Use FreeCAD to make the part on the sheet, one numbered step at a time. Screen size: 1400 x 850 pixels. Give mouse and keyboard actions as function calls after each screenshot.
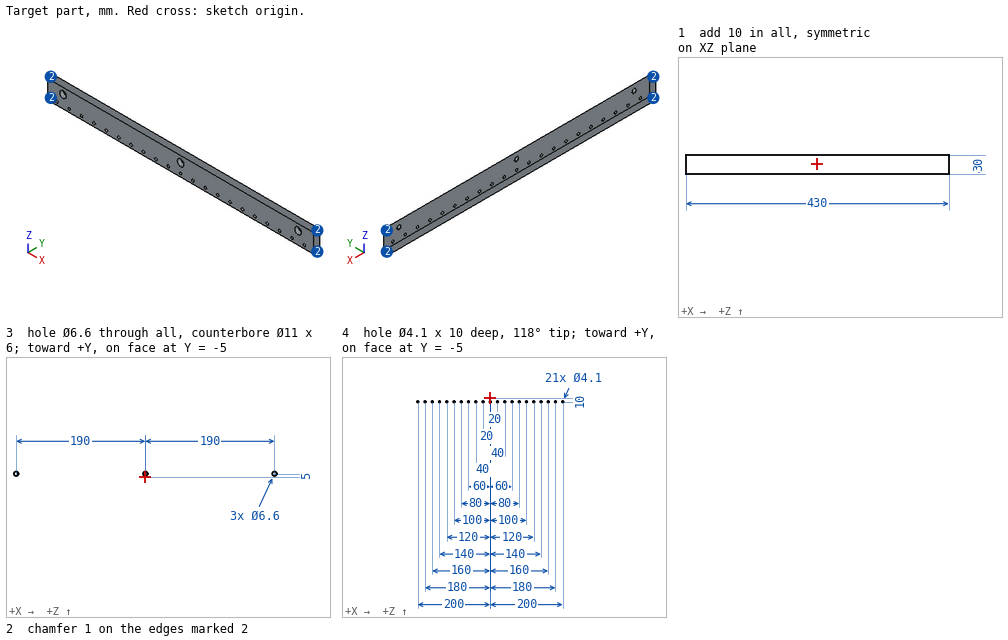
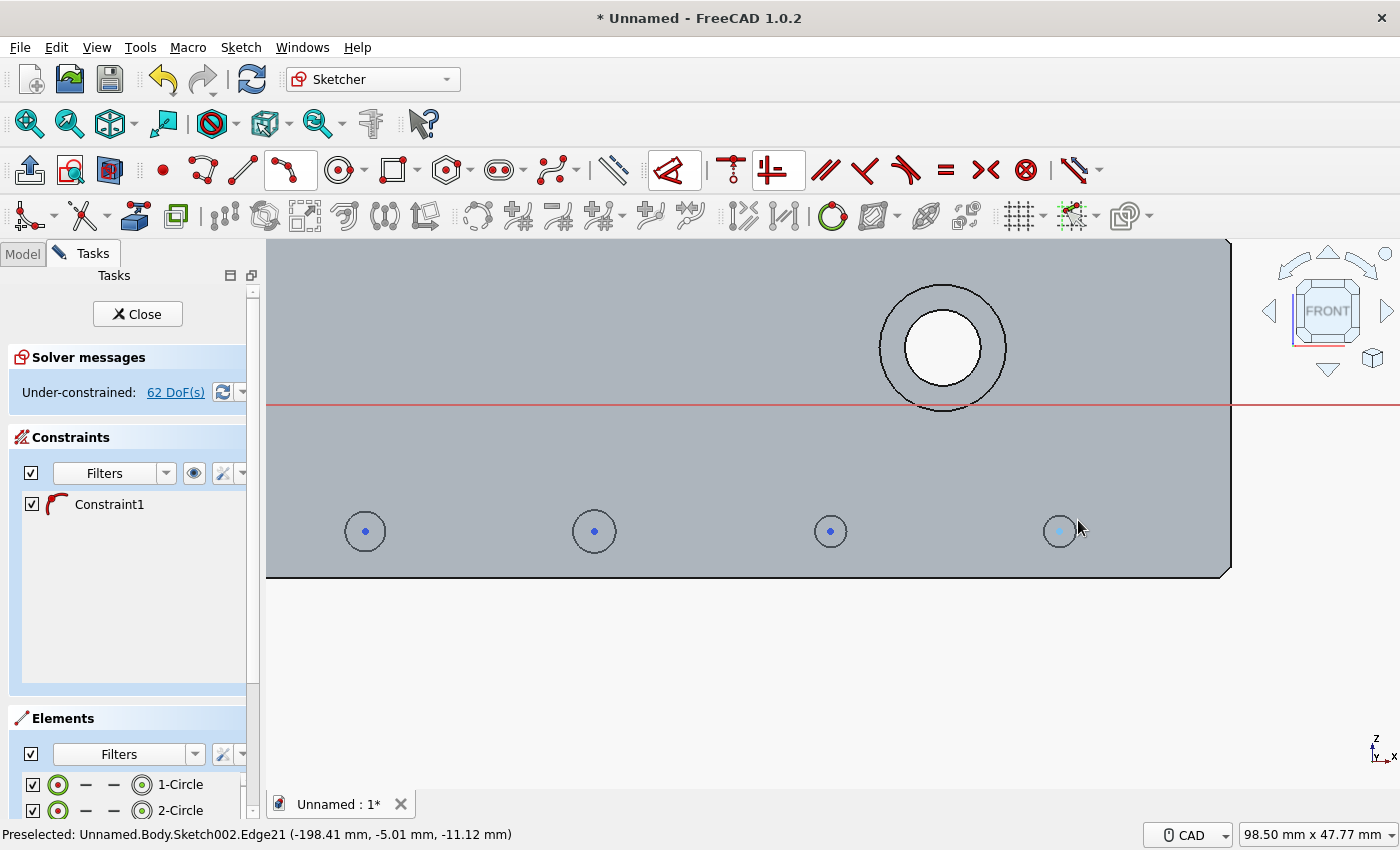
click(1071, 520)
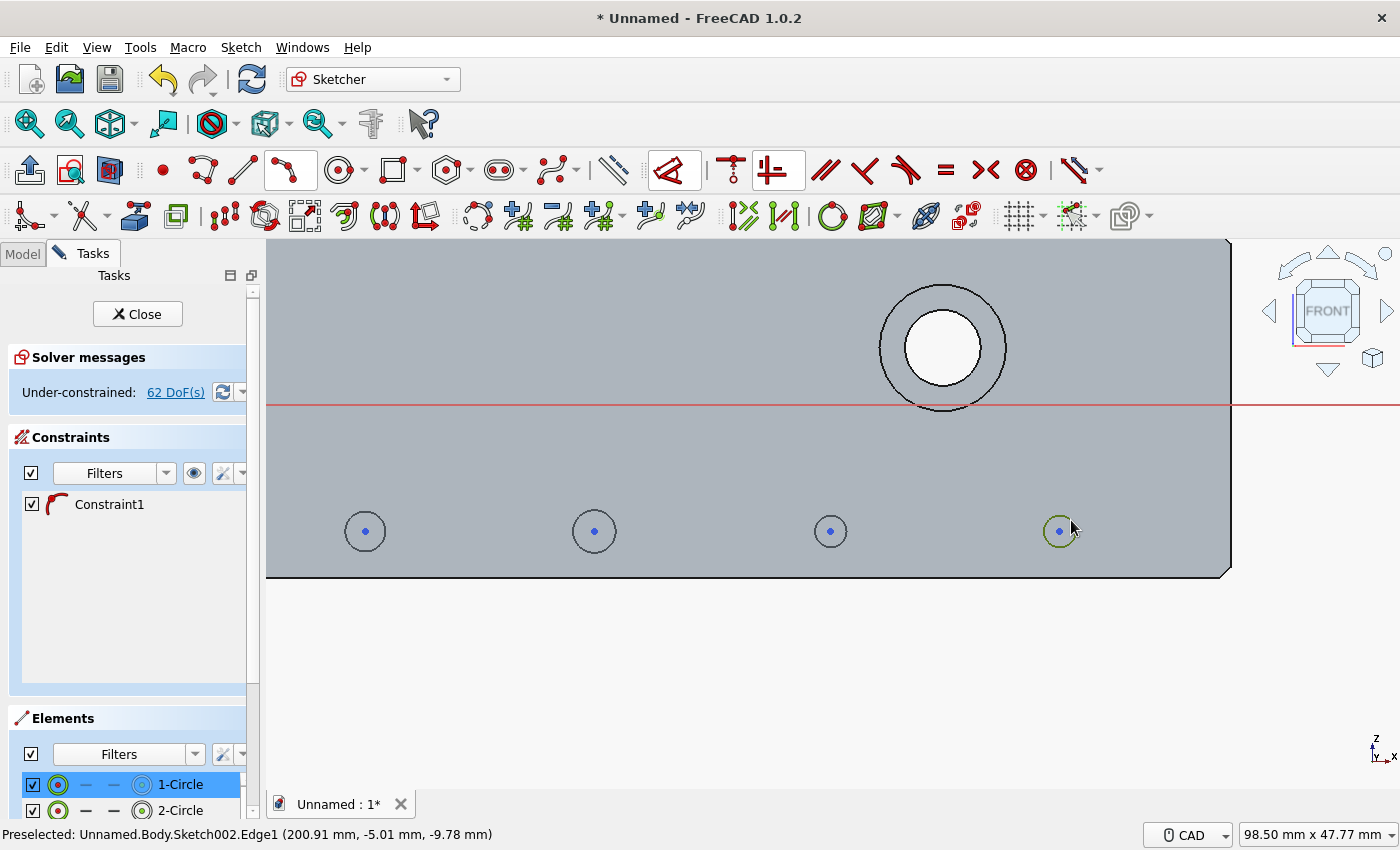
click(842, 520)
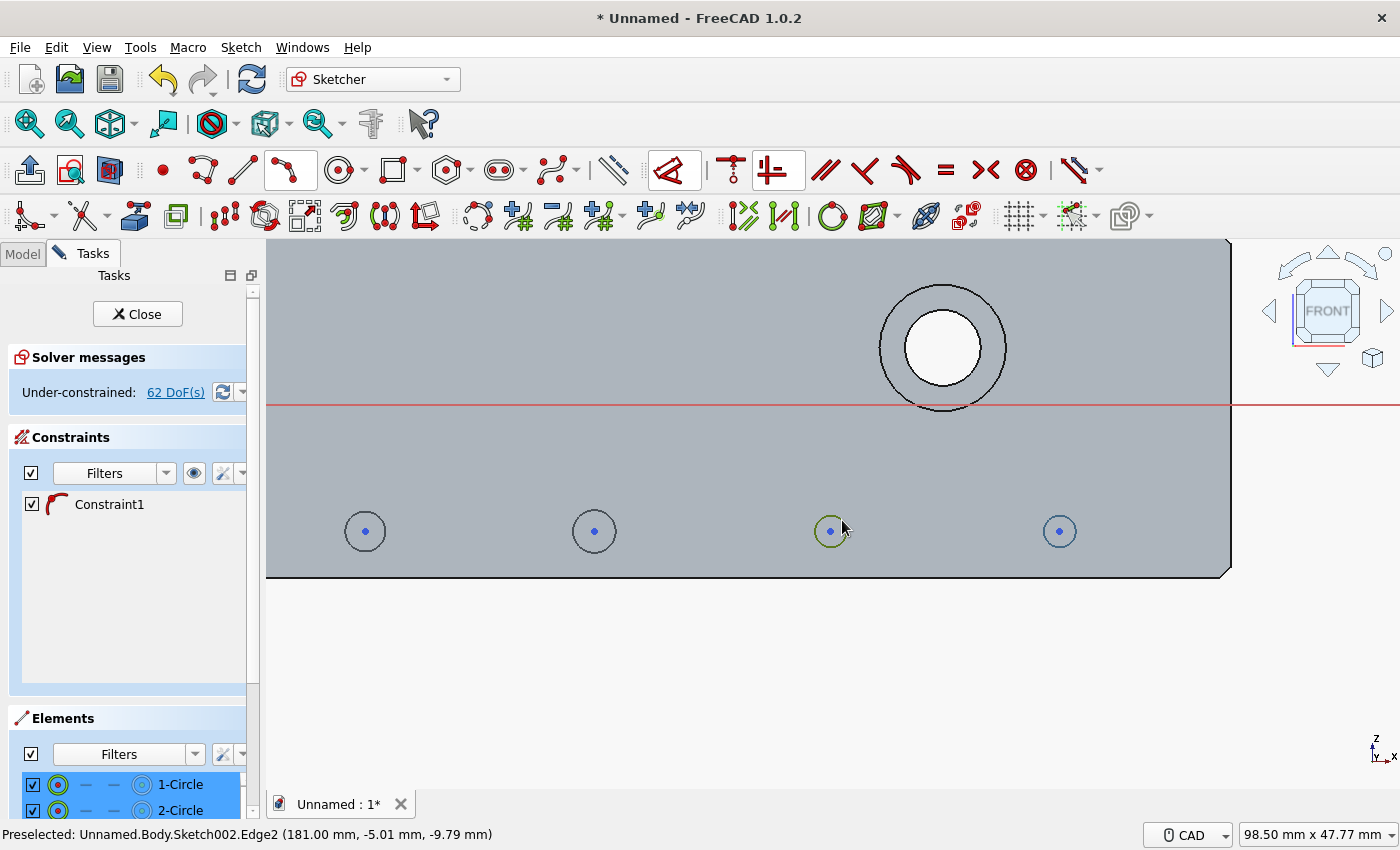
click(609, 516)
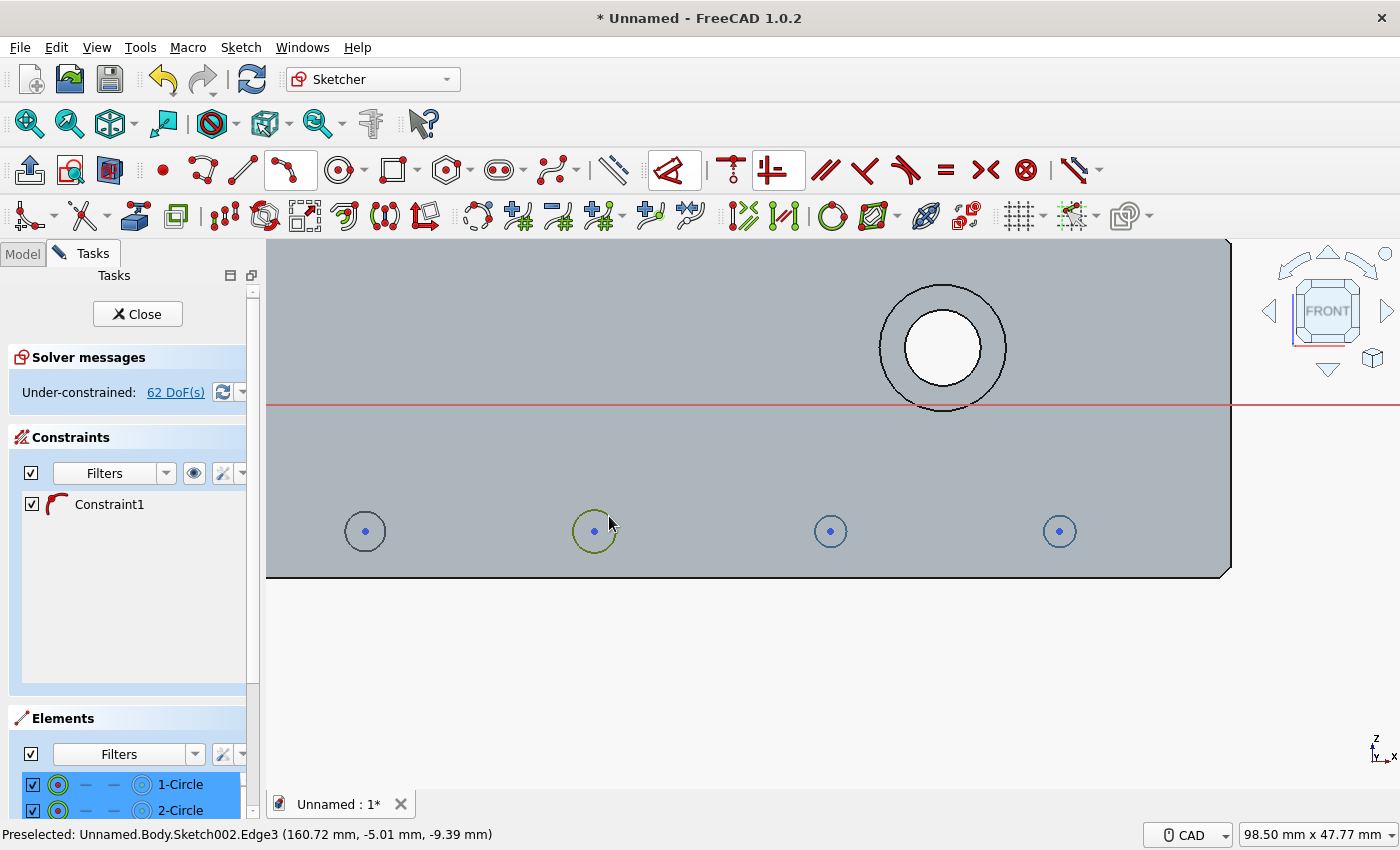
click(379, 517)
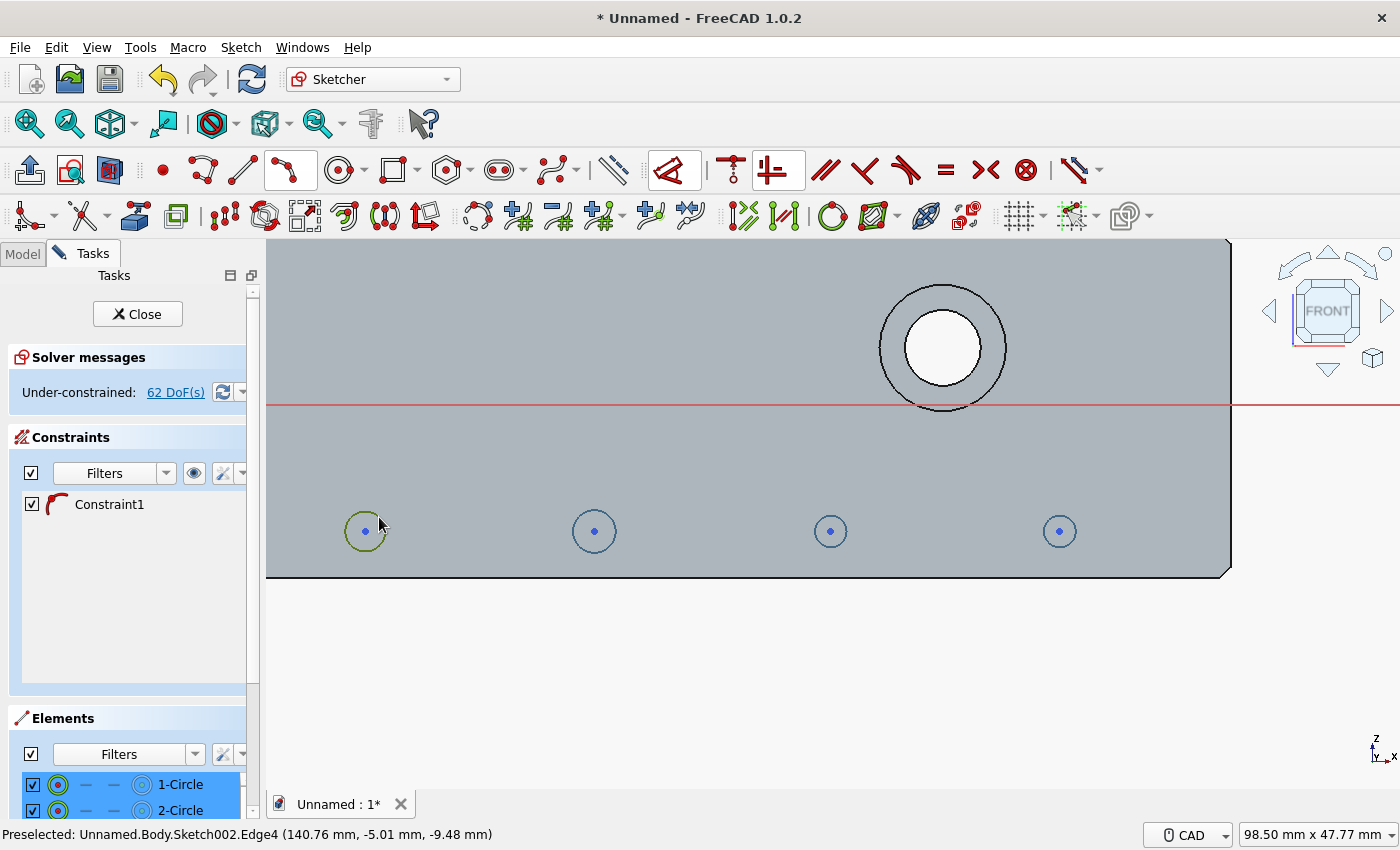
scroll(1079, 520, down, 10)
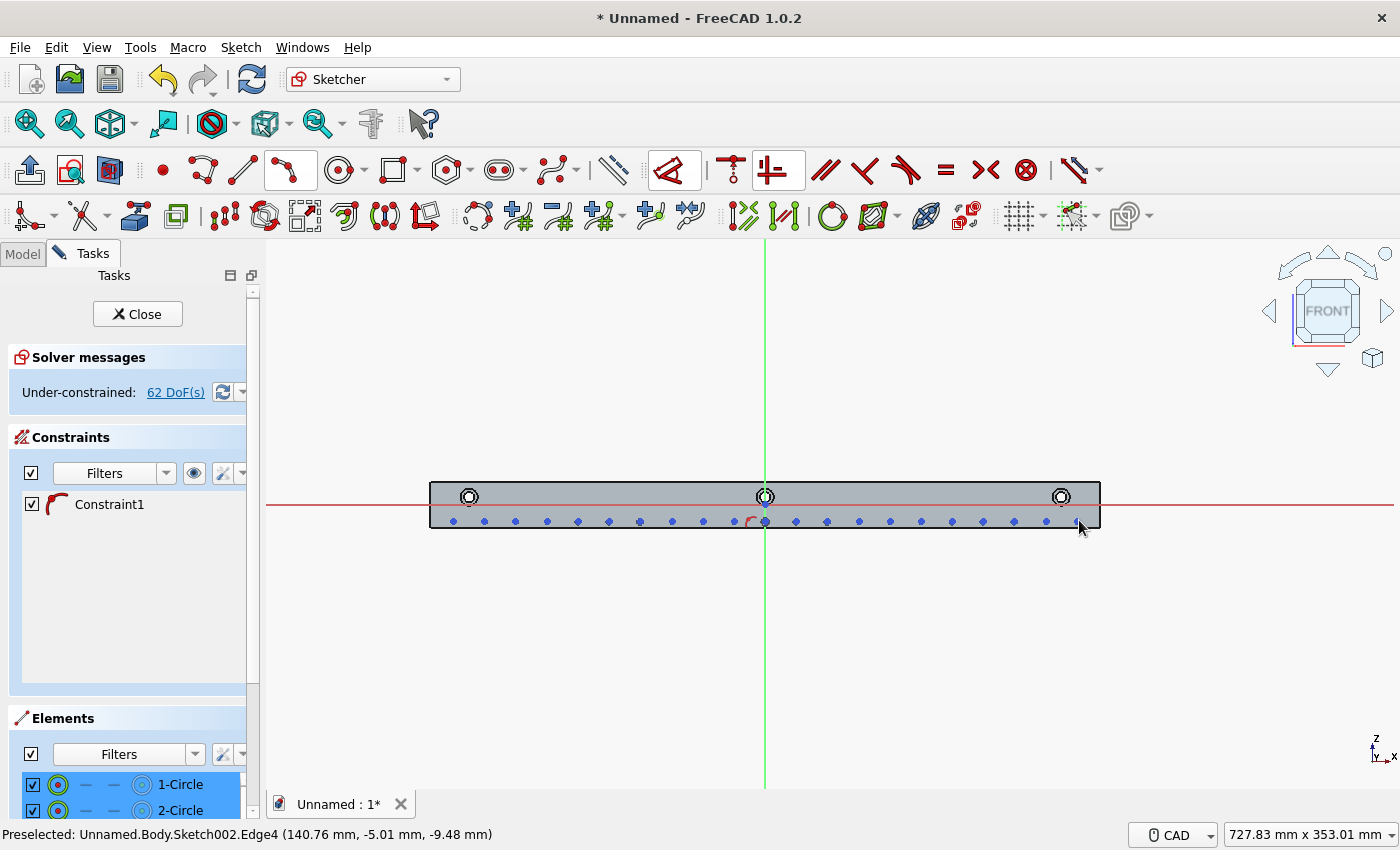
scroll(954, 520, up, 9)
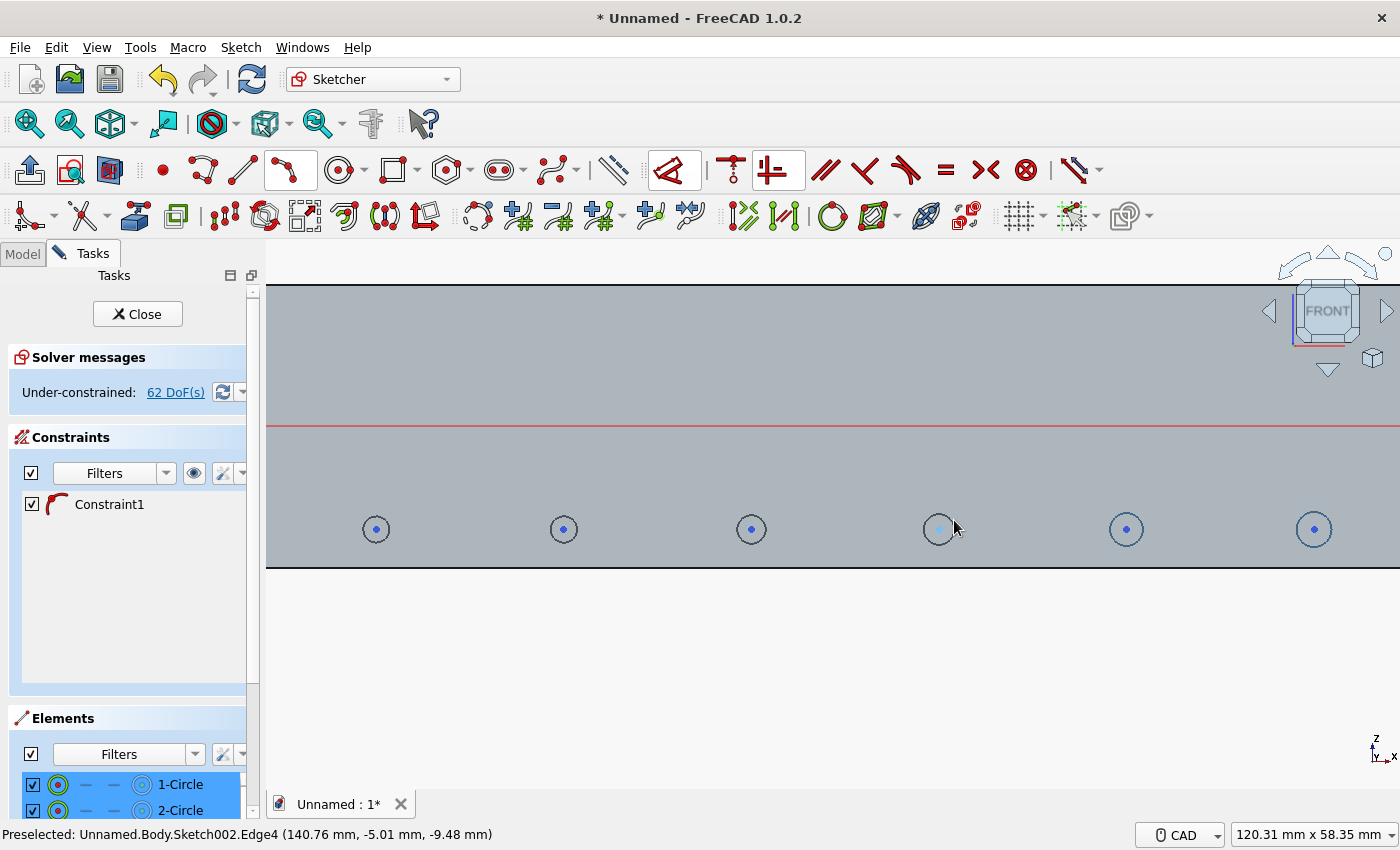
click(950, 519)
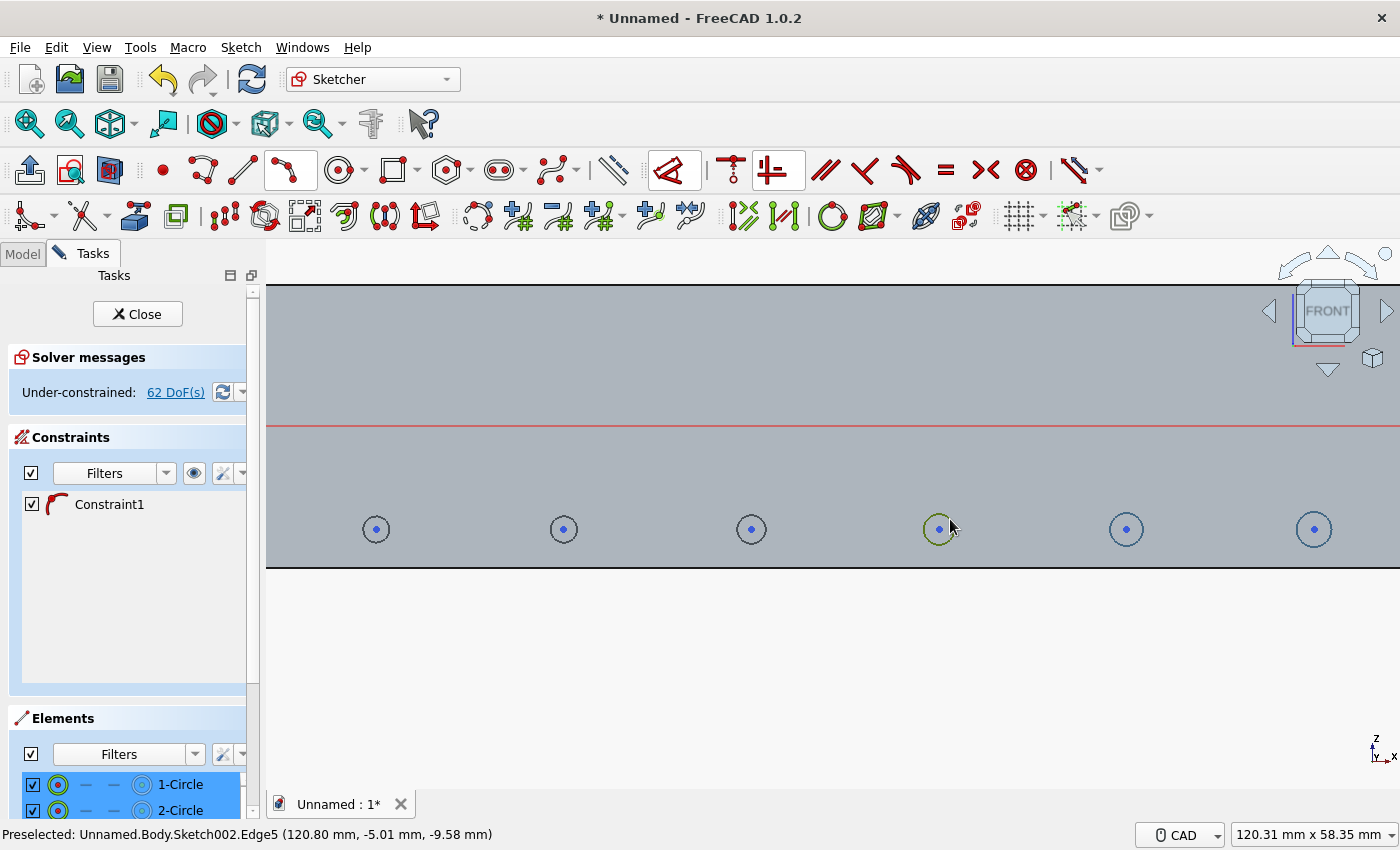
click(761, 519)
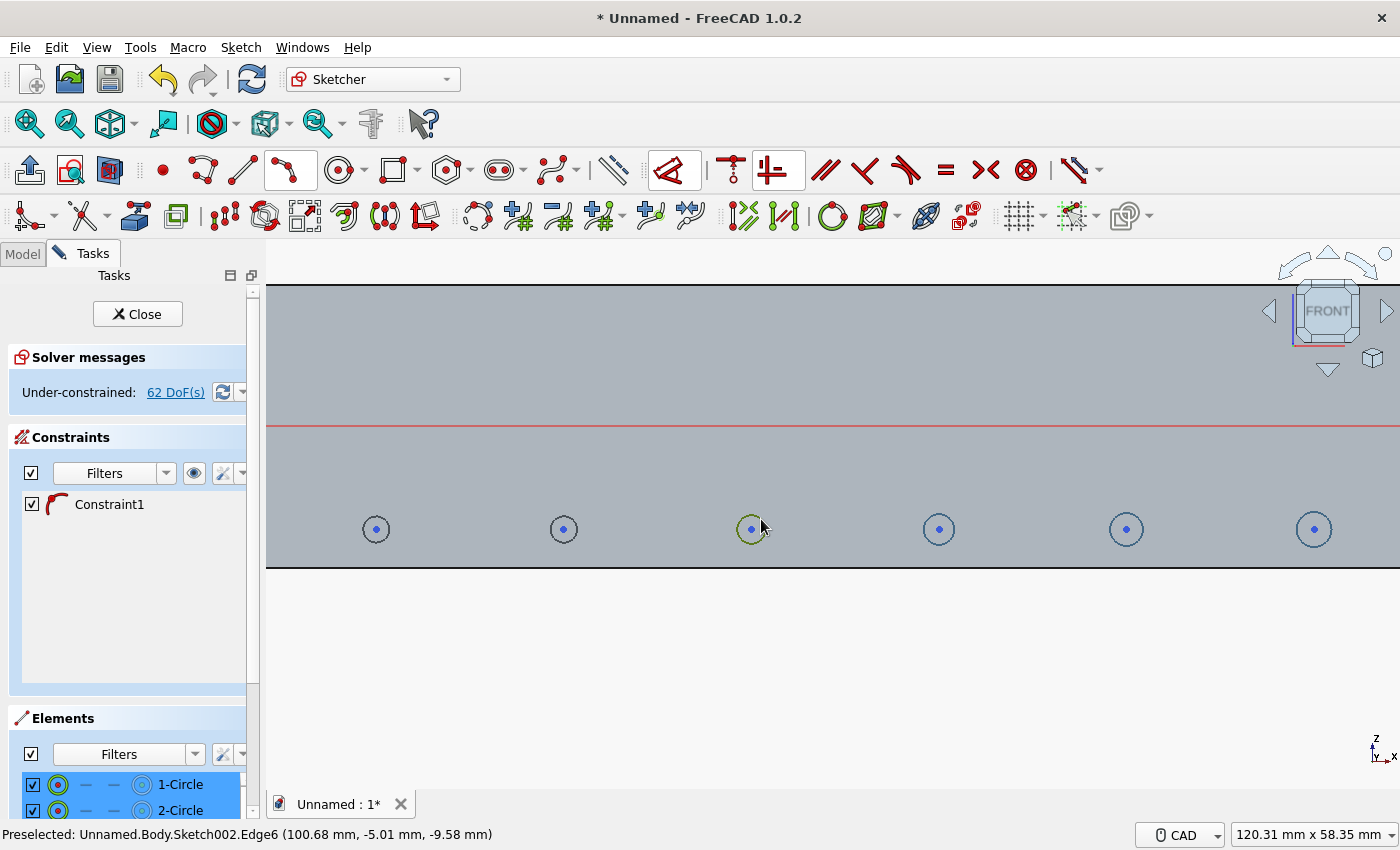
click(573, 520)